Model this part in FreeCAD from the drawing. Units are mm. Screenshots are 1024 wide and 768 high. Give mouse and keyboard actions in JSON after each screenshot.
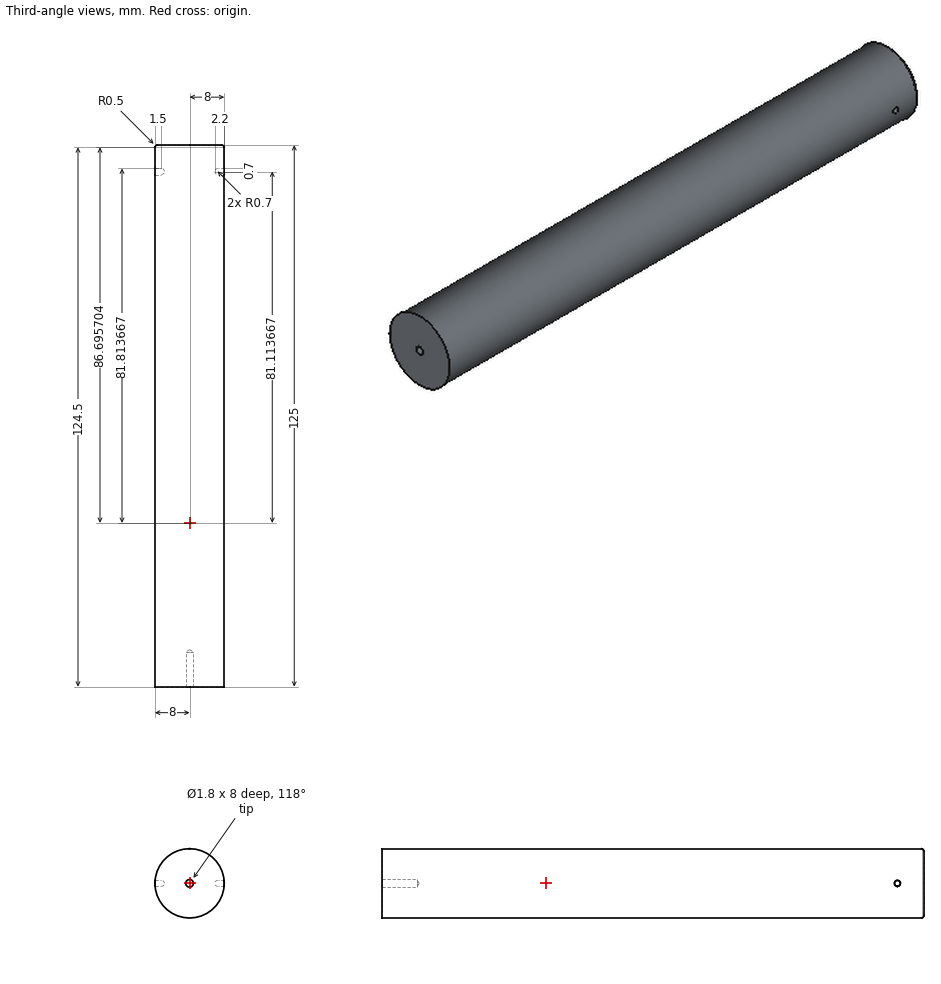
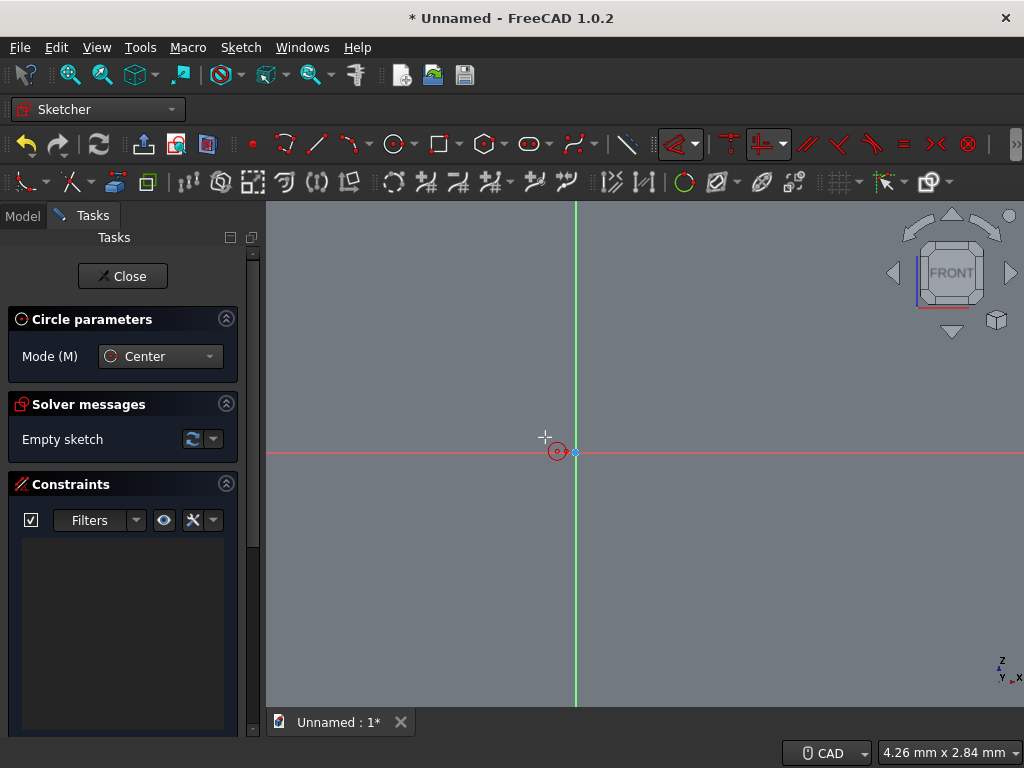
{"action": "left_click", "coordinate": [576, 453]}
{"action": "left_click", "coordinate": [689, 340]}
{"action": "key", "text": "Escape"}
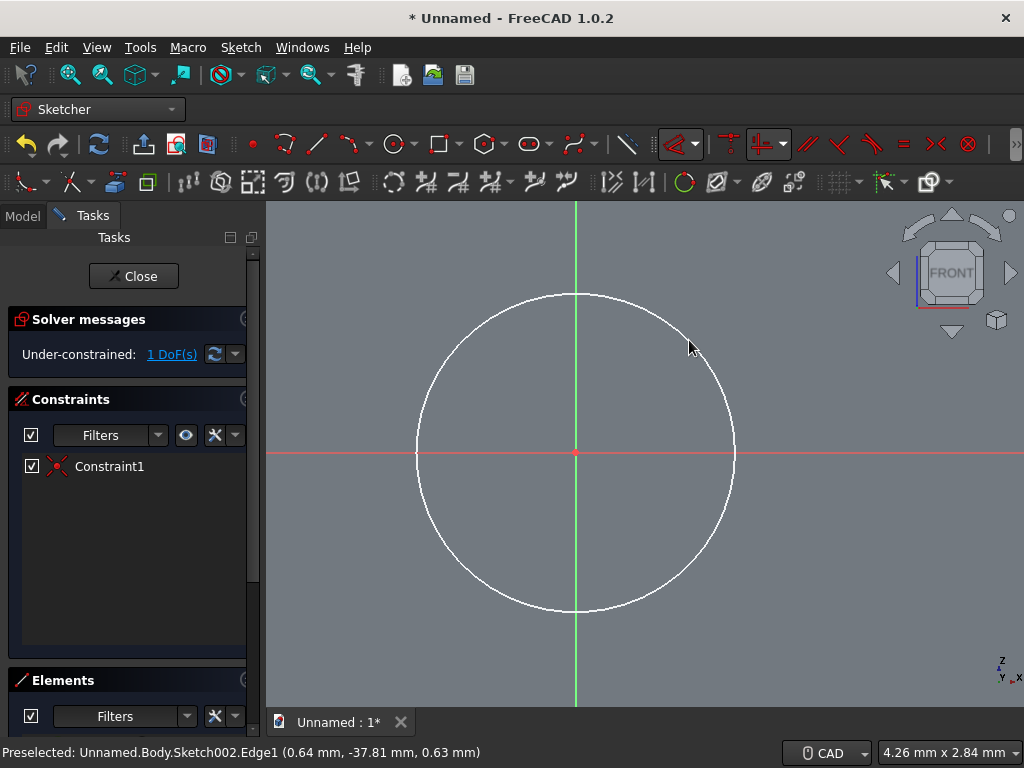
{"action": "left_click", "coordinate": [688, 340]}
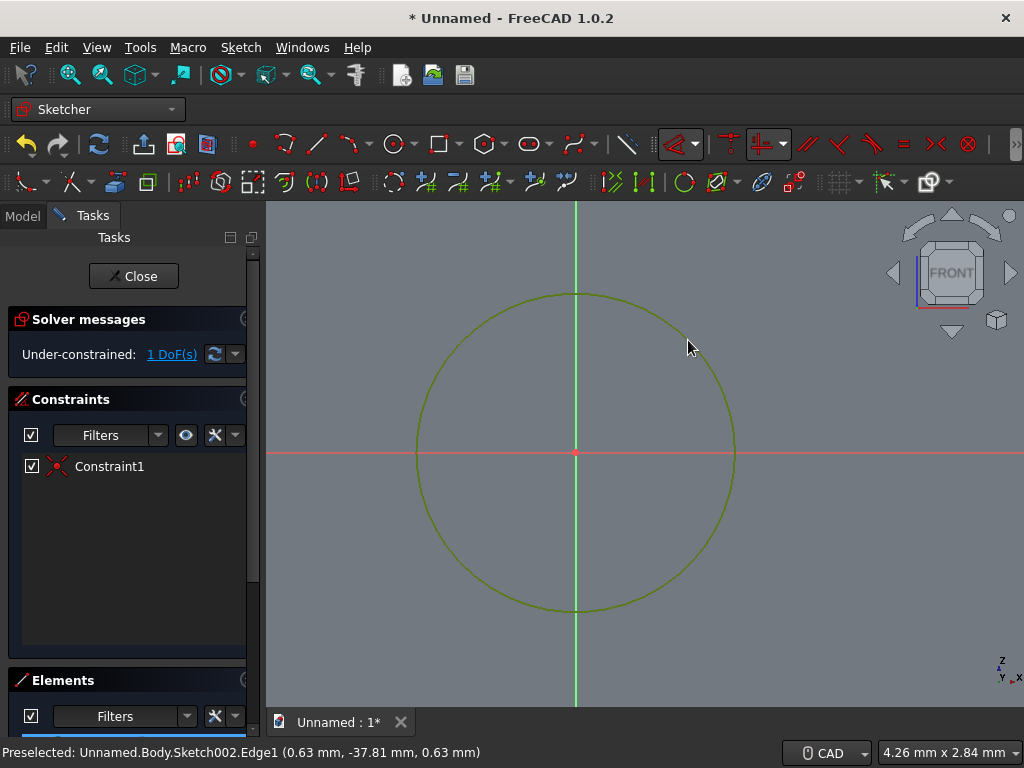
{"action": "key", "text": "k o"}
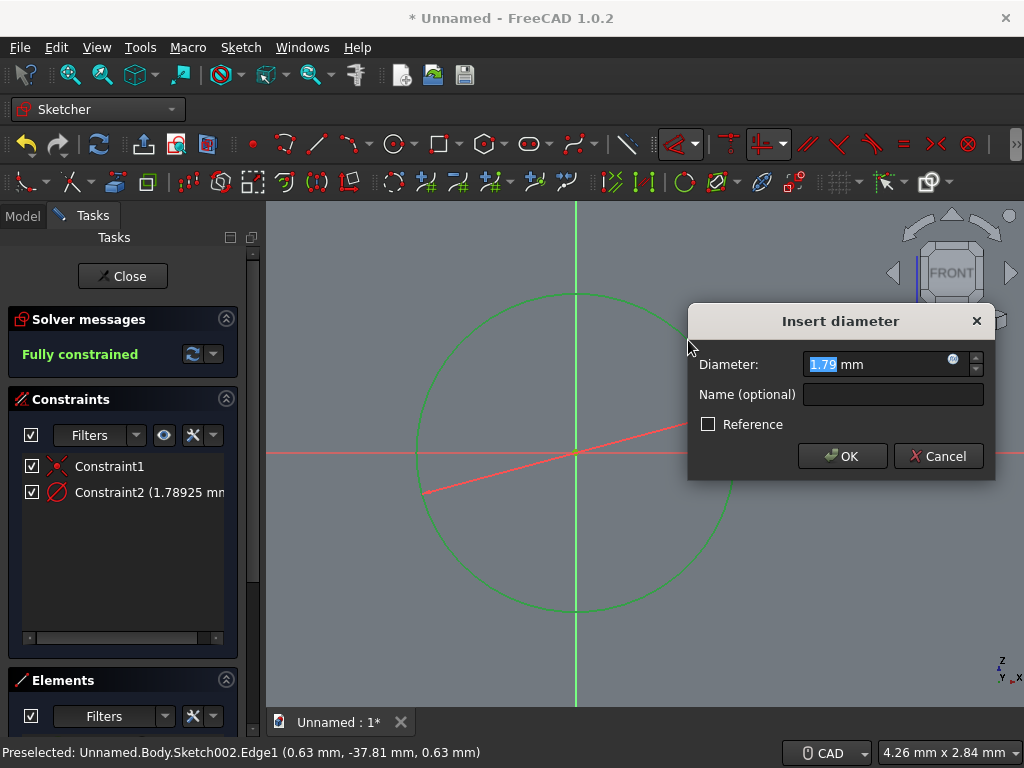
{"action": "type", "text": "1.8"}
{"action": "key", "text": "Return"}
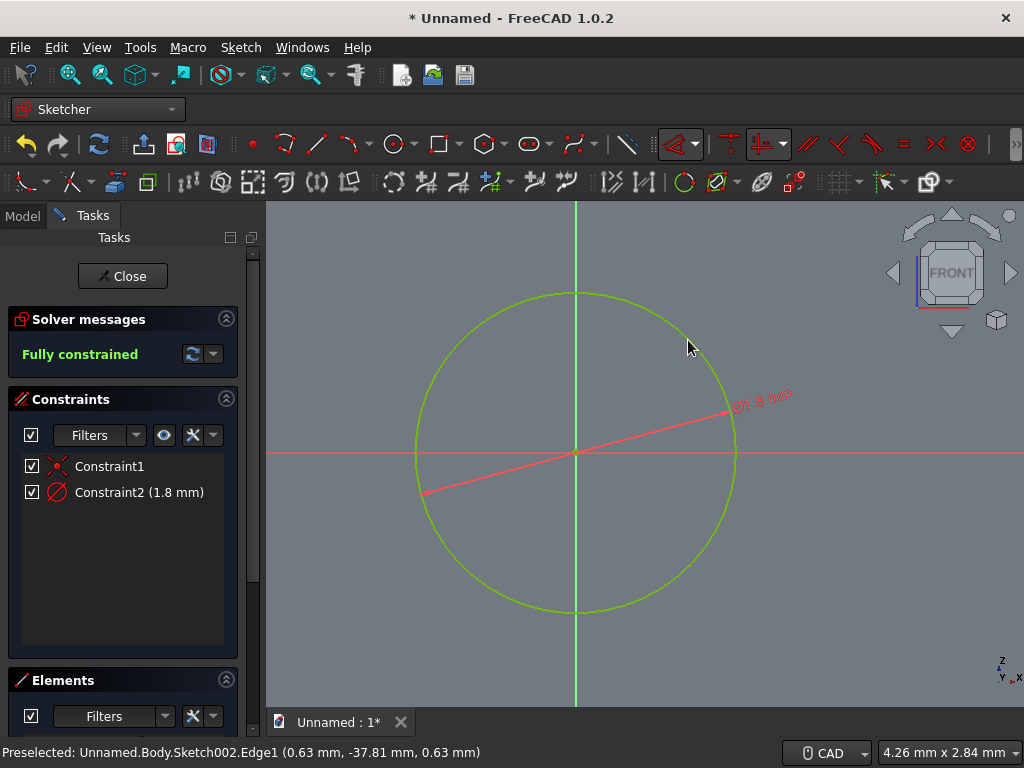
{"action": "left_click", "coordinate": [123, 276]}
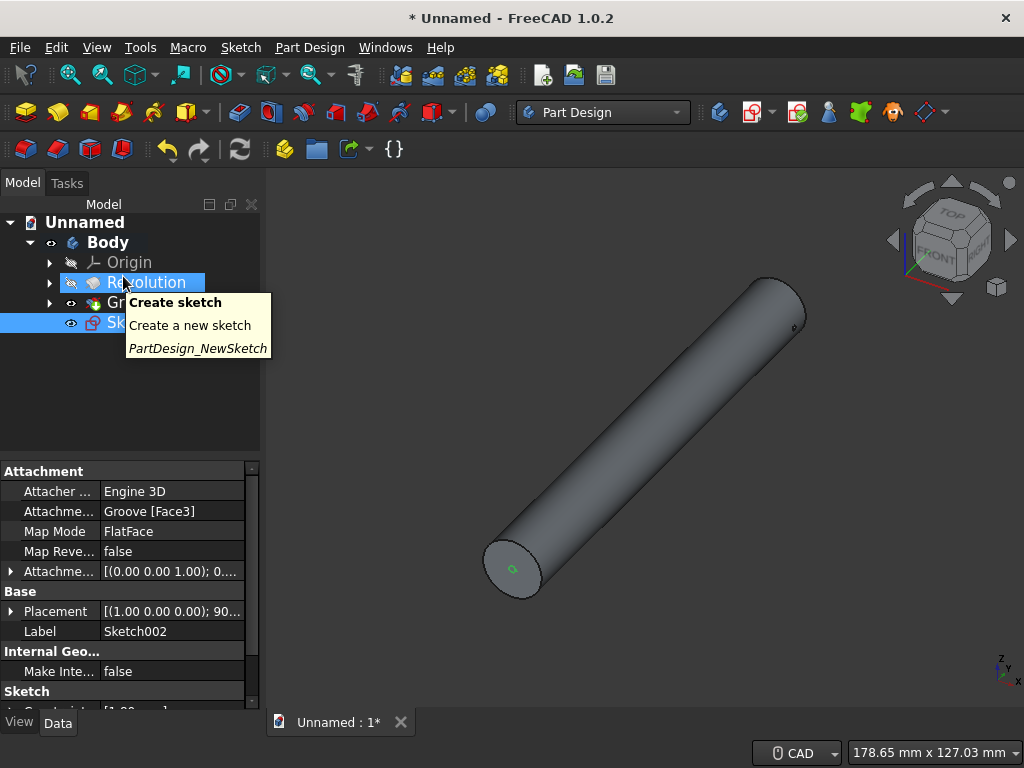
{"action": "left_click", "coordinate": [272, 112]}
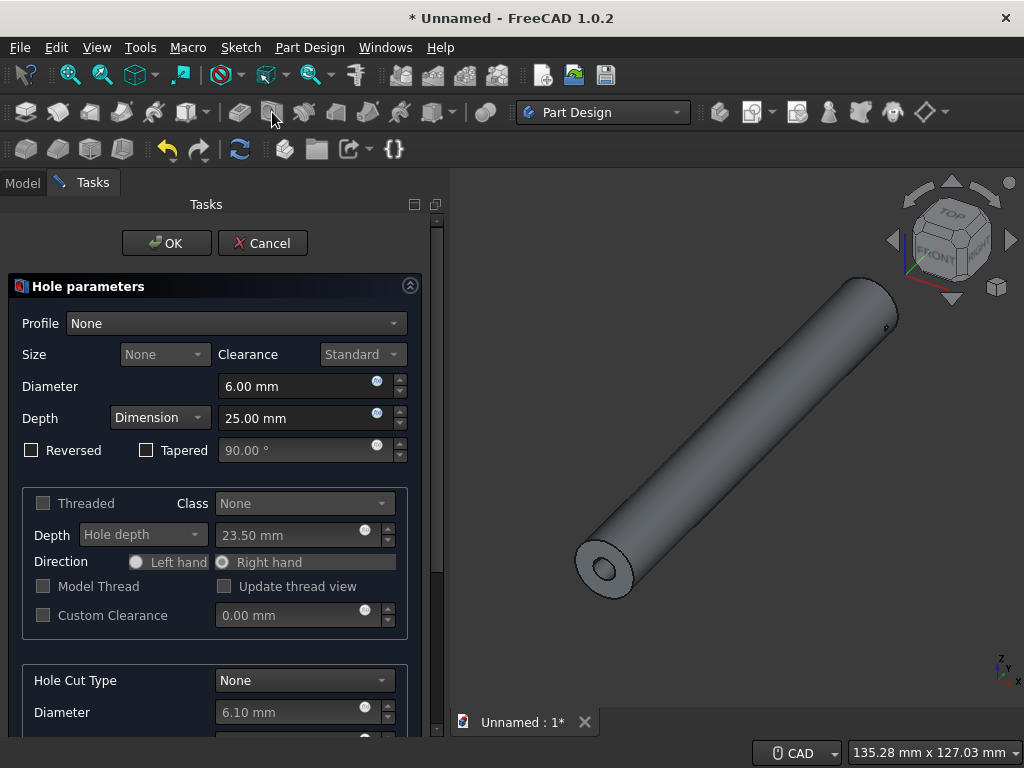
{"action": "triple_click", "coordinate": [305, 386]}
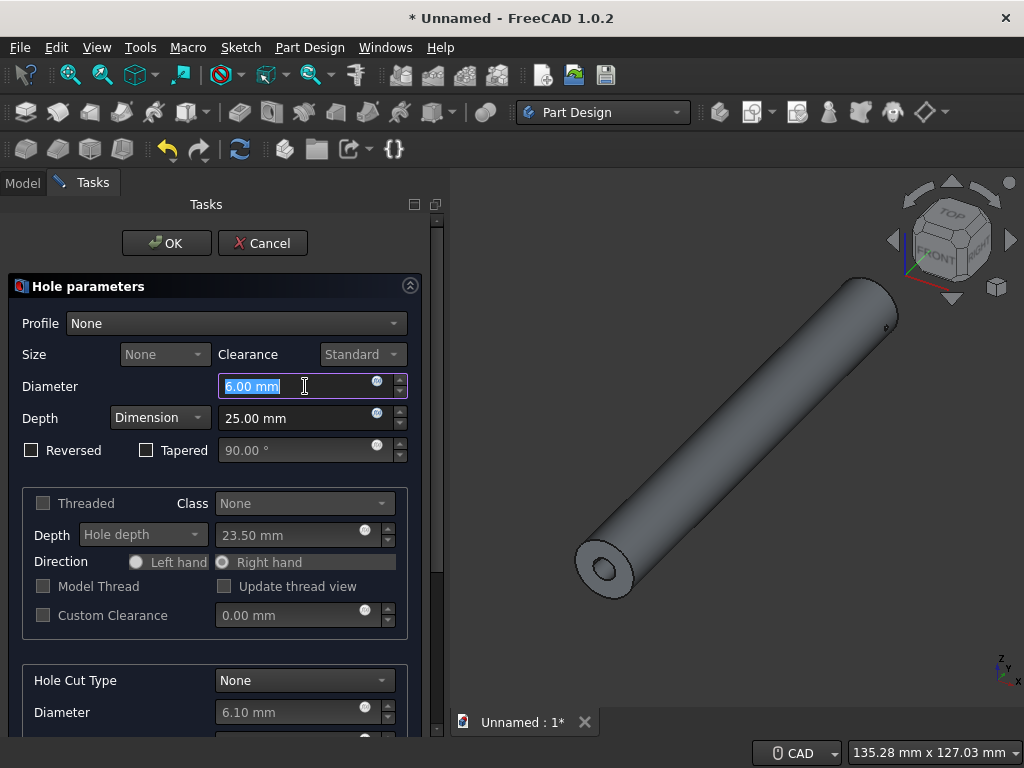
{"action": "type", "text": "1.8"}
{"action": "key", "text": "Tab"}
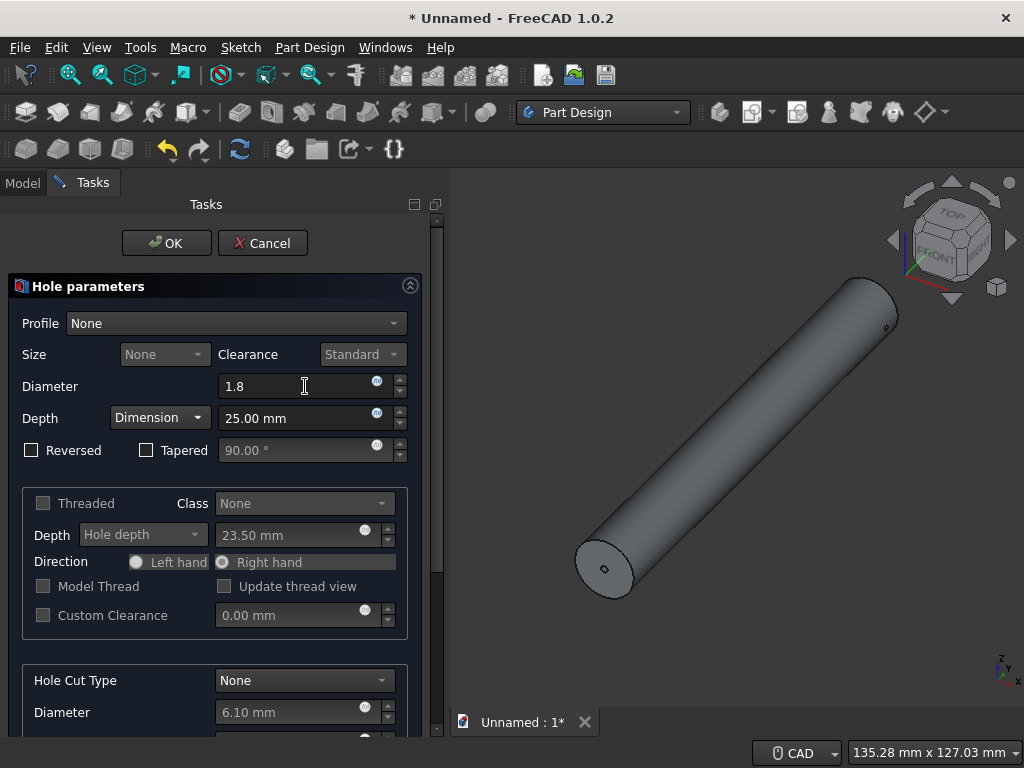
{"action": "triple_click", "coordinate": [305, 418]}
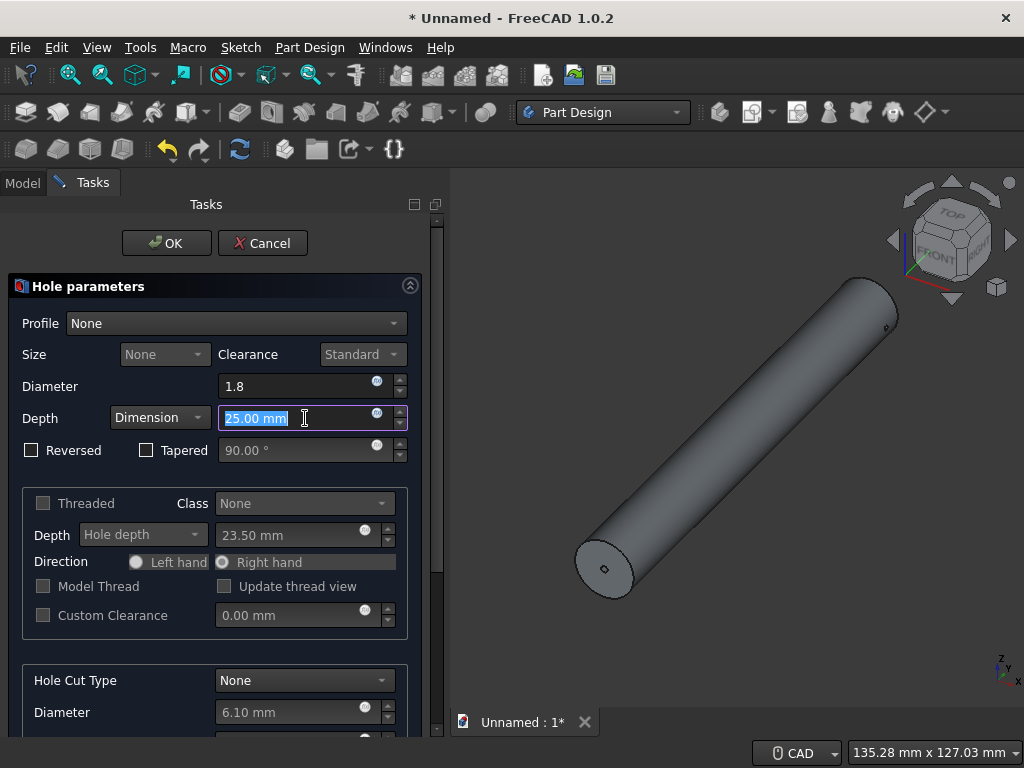
{"action": "type", "text": "8"}
{"action": "key", "text": "Tab"}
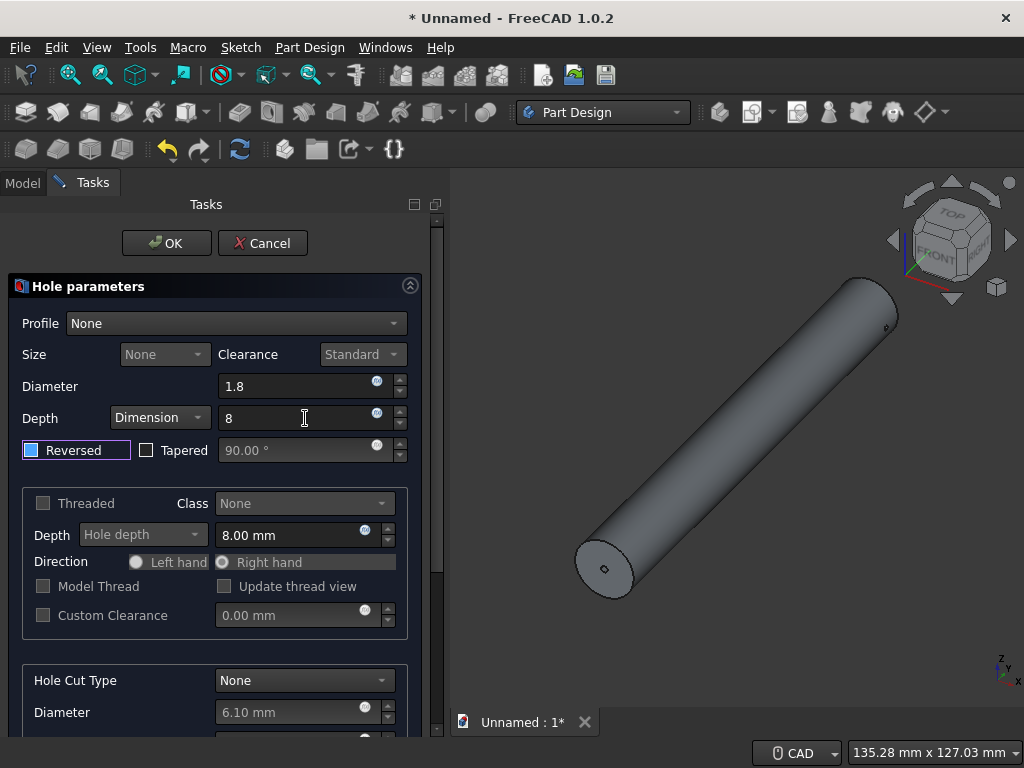
{"action": "left_click", "coordinate": [167, 243]}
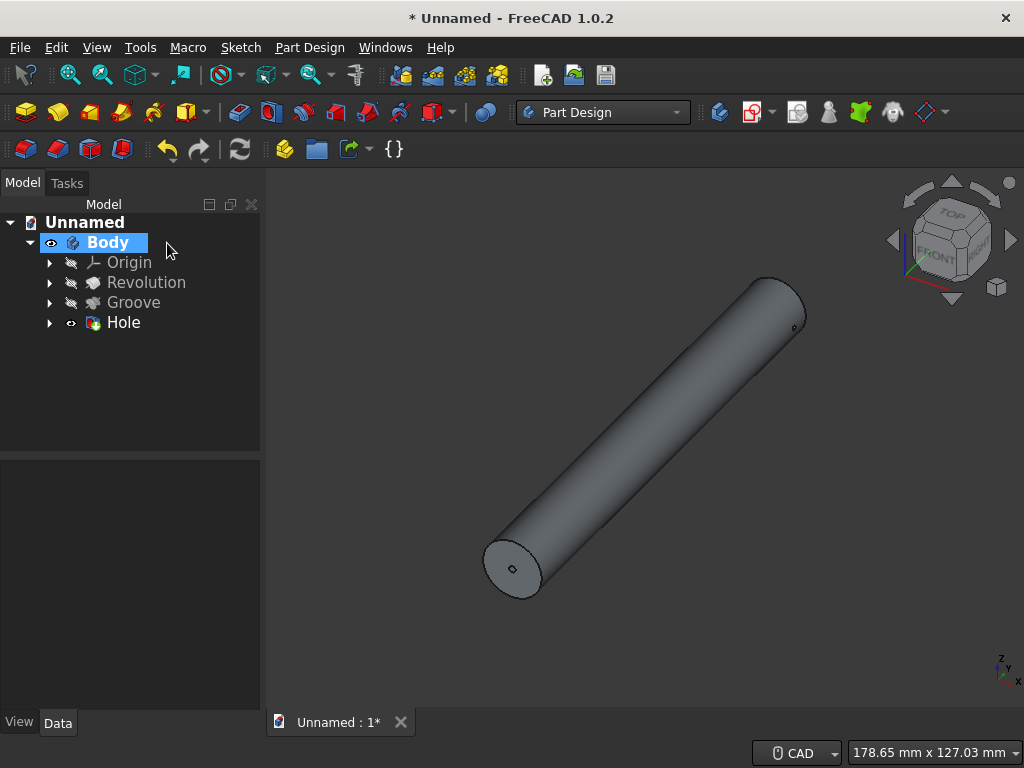
{"action": "key", "text": "0"}